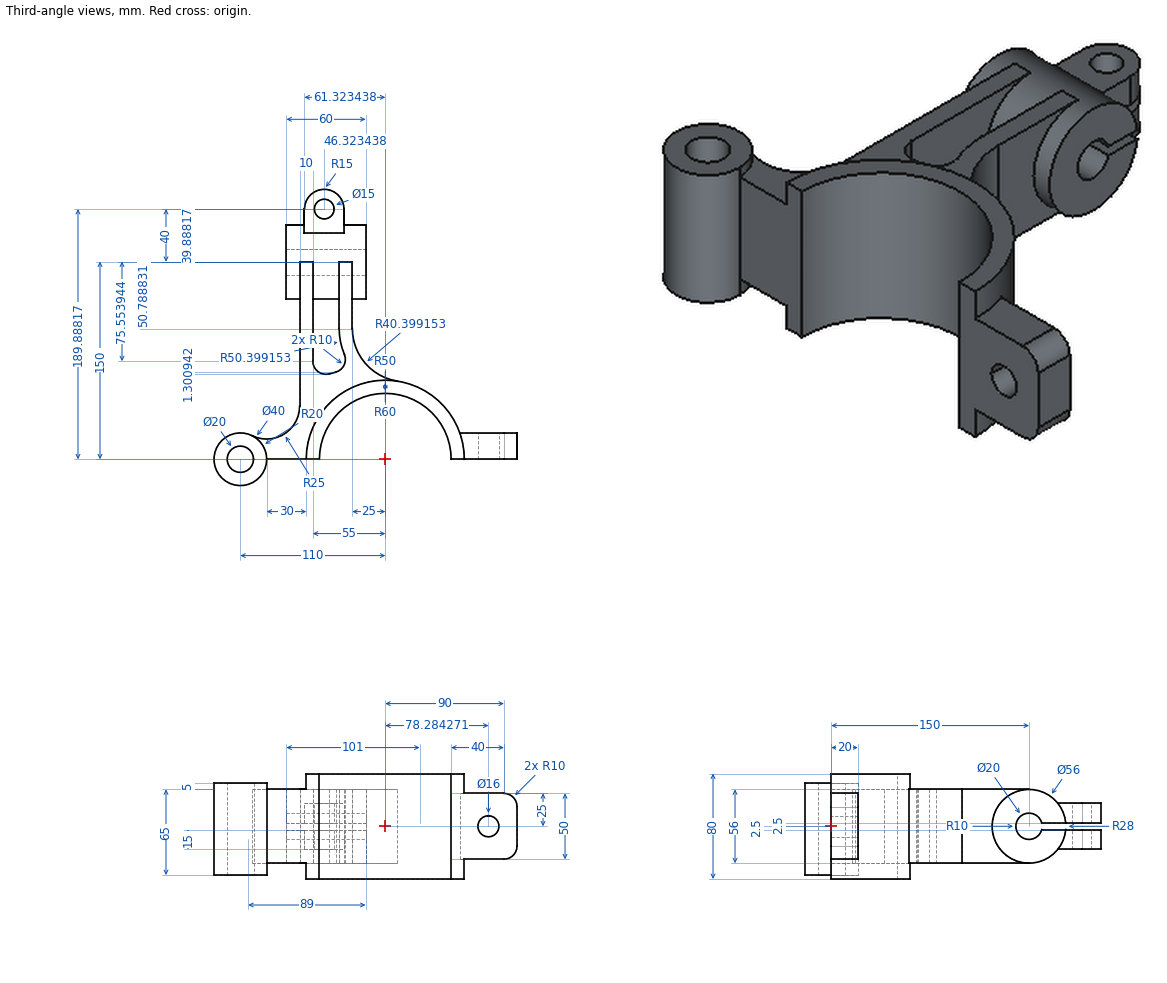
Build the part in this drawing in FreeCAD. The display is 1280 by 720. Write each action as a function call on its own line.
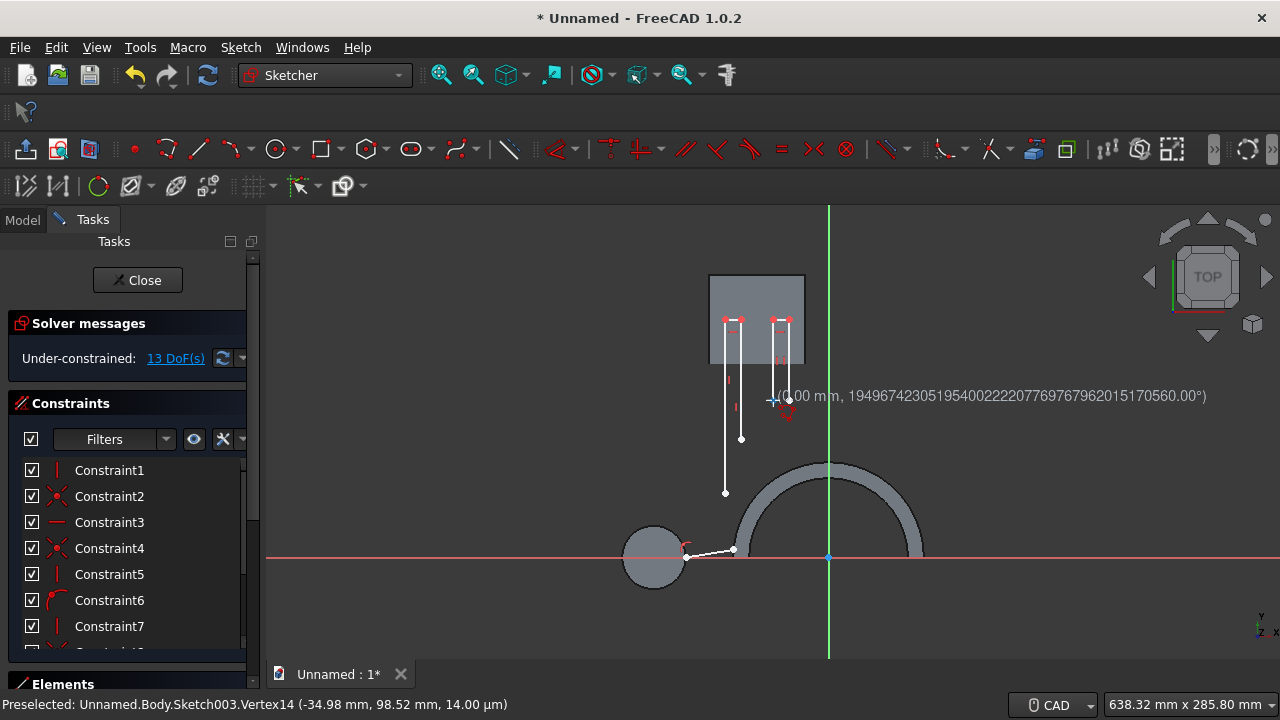
click(200, 150)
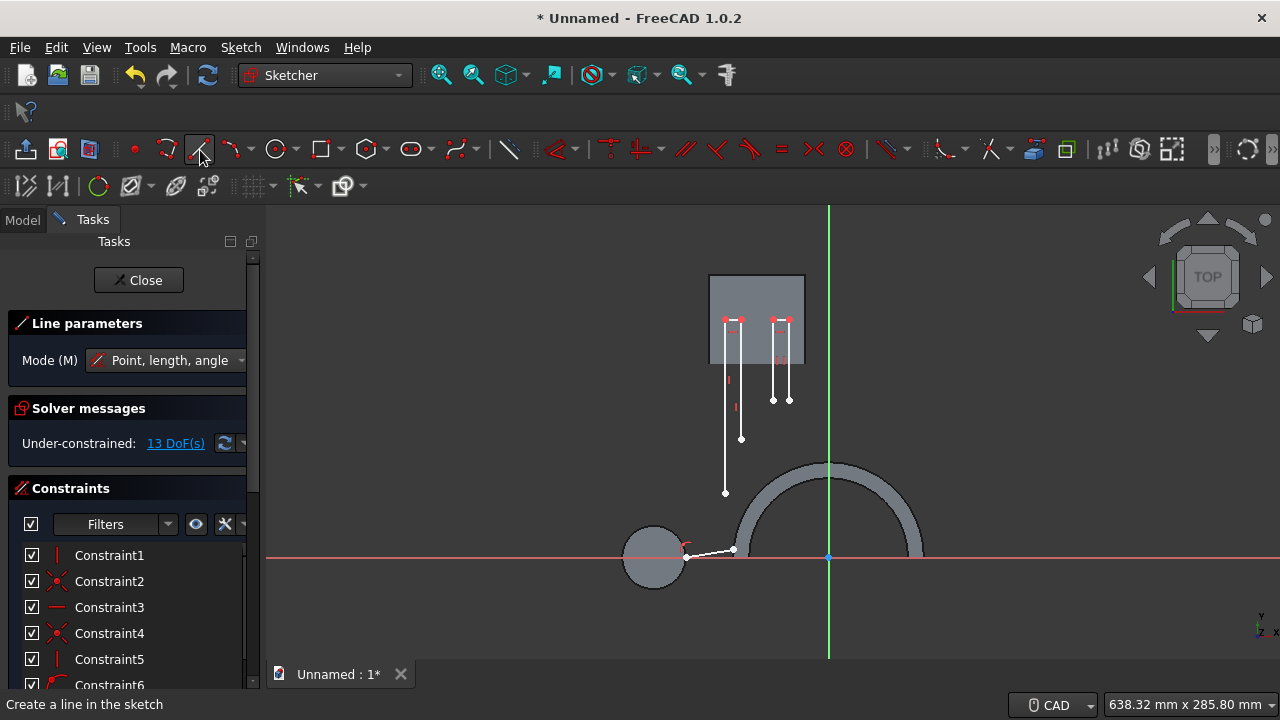
click(769, 452)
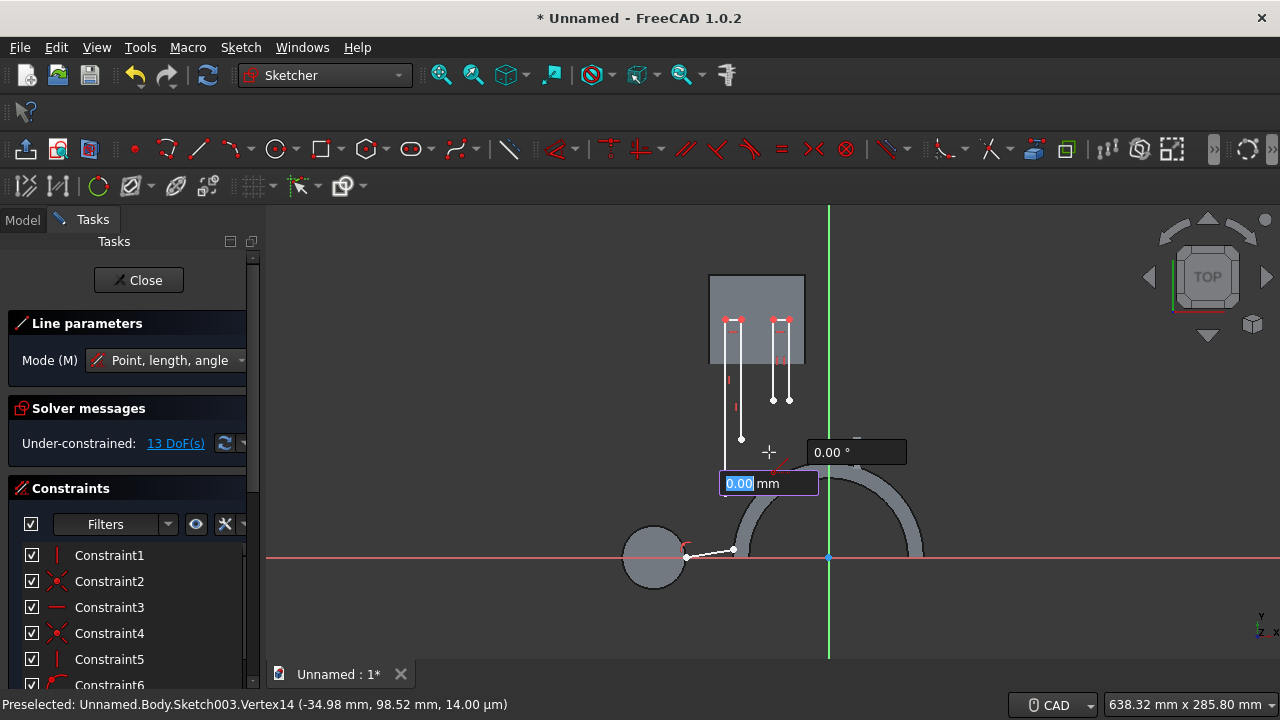
scroll(761, 455, up, 4)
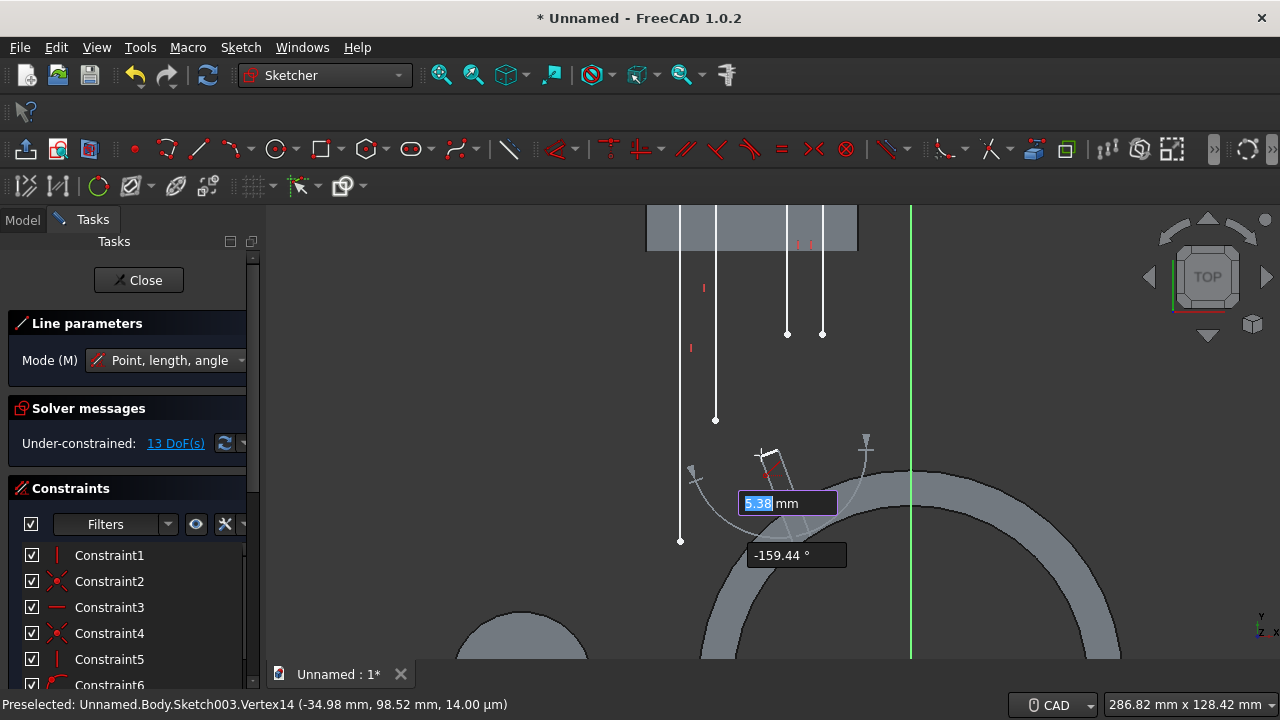
click(761, 453)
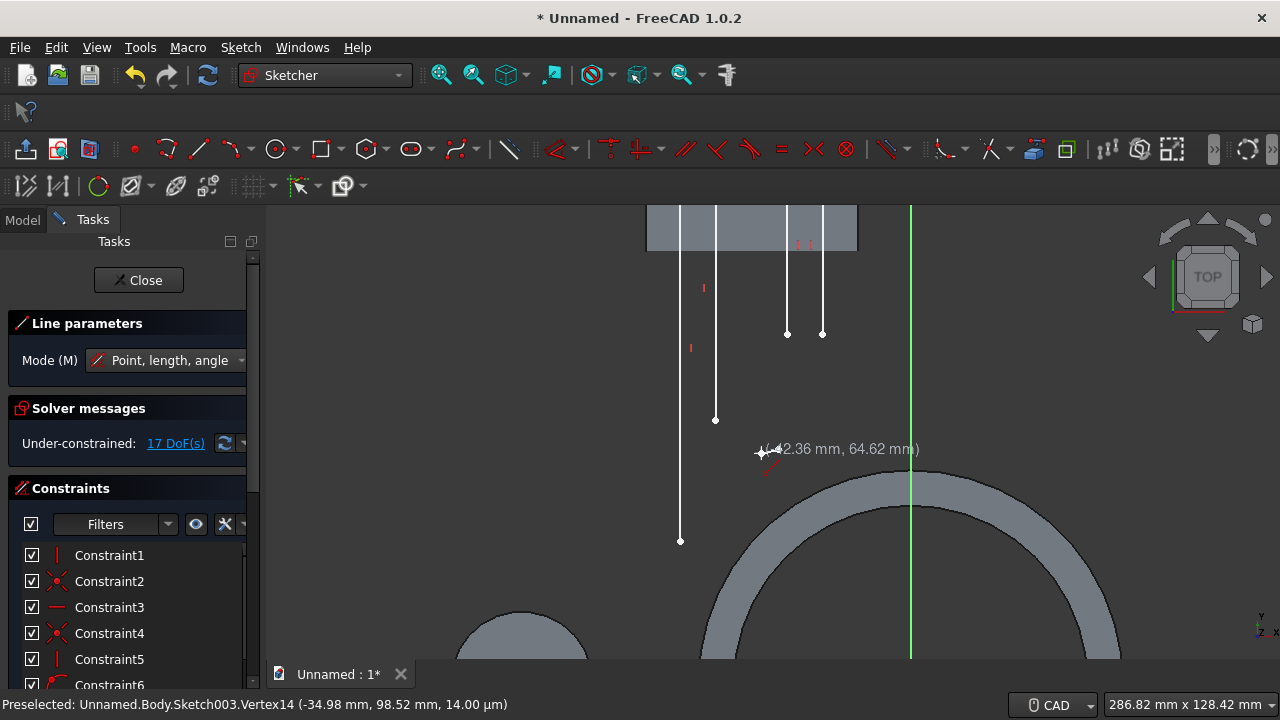
key(g)
key(3)
key(a)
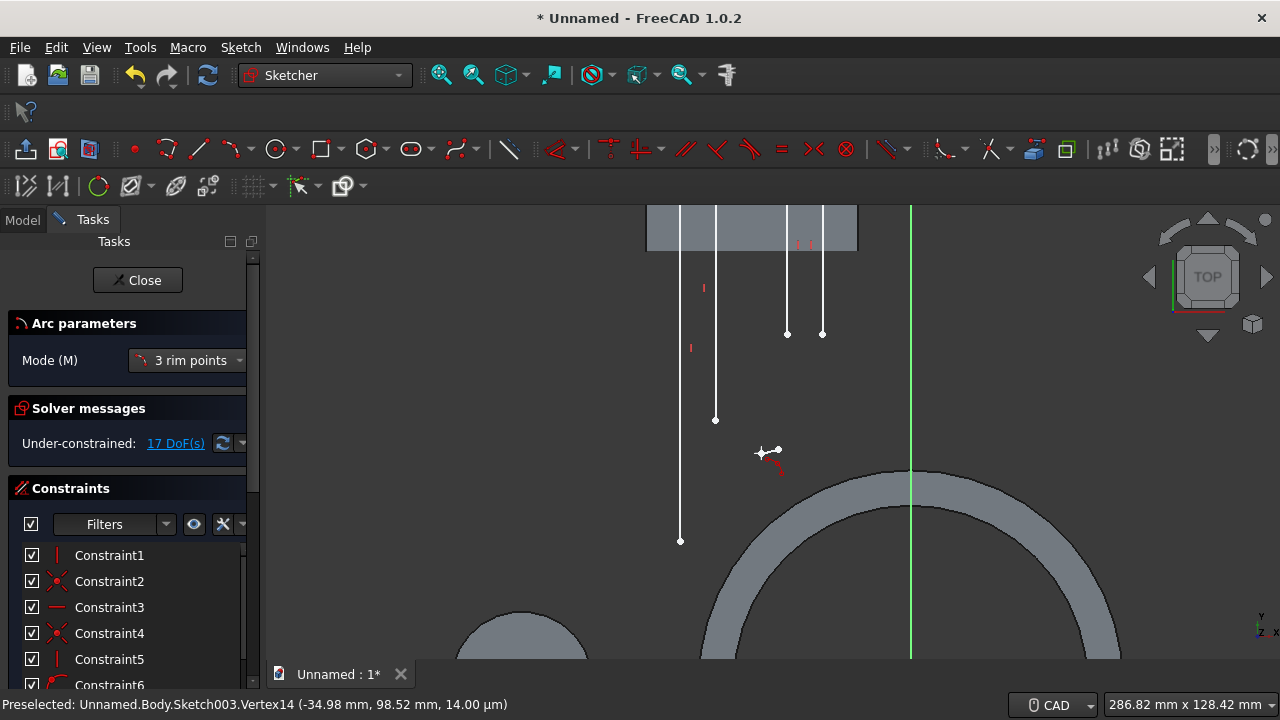
click(680, 541)
click(553, 619)
click(639, 615)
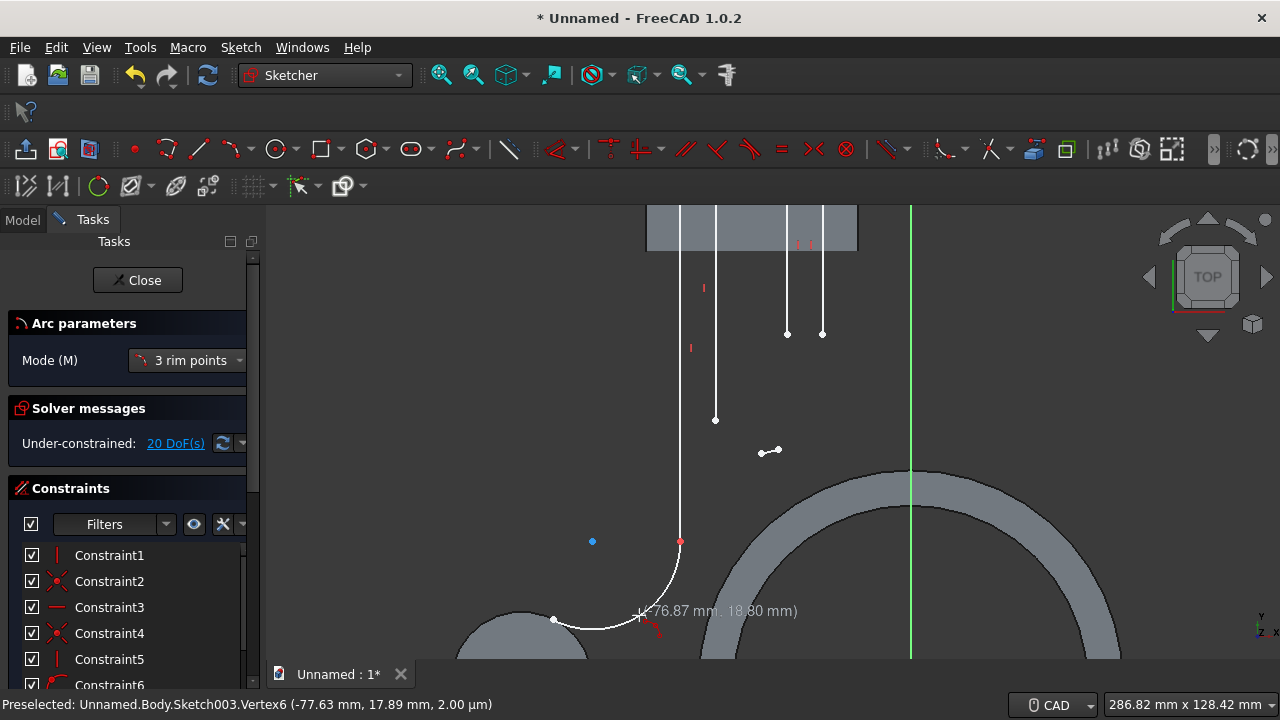
click(553, 620)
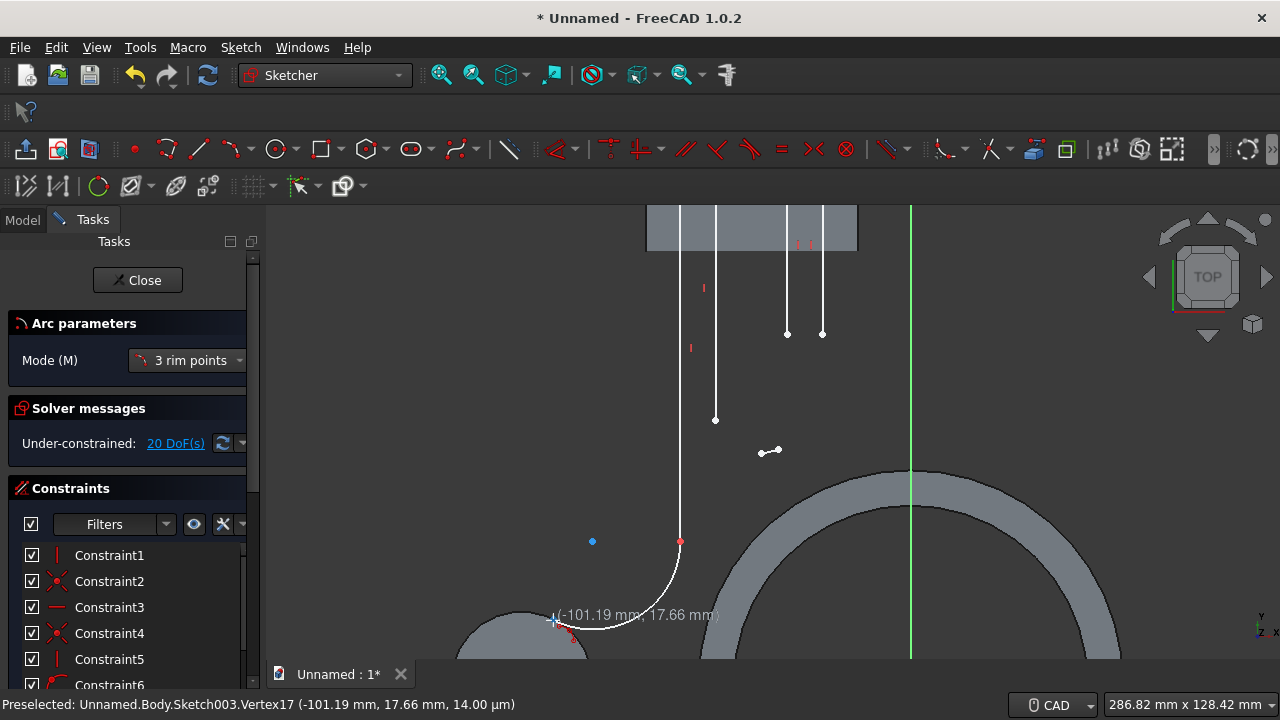
scroll(651, 450, down, 3)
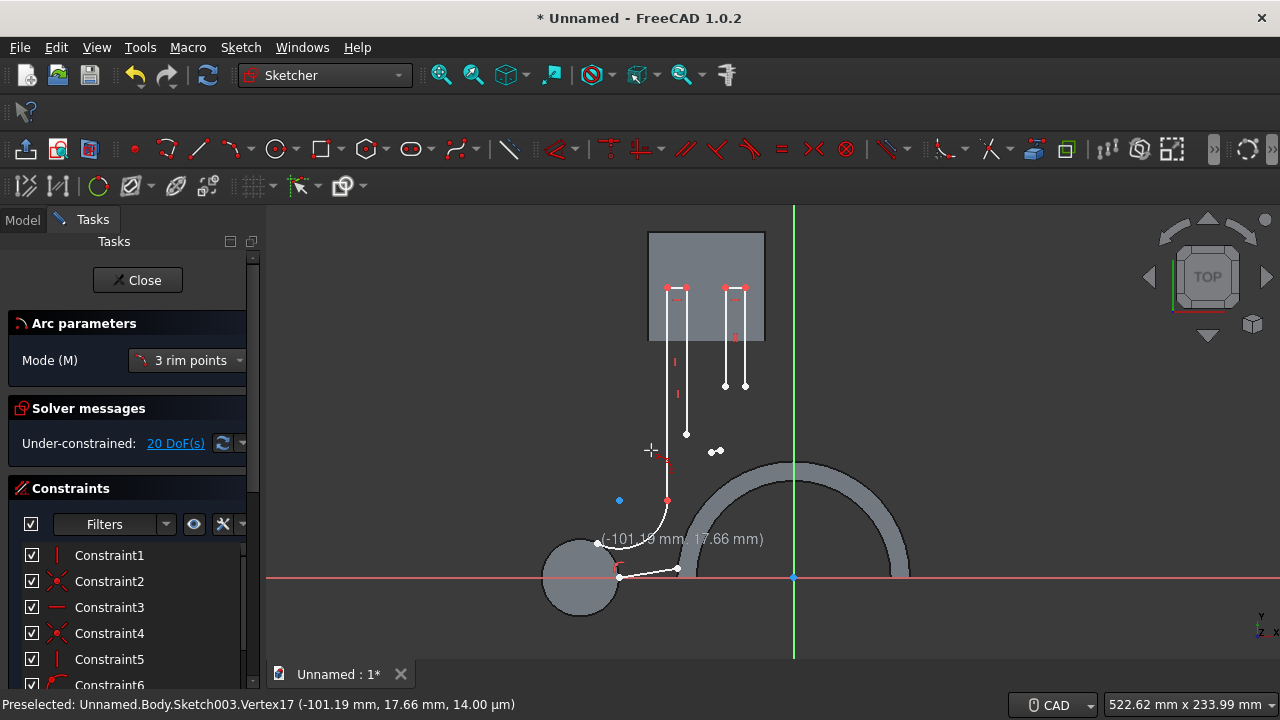
click(620, 578)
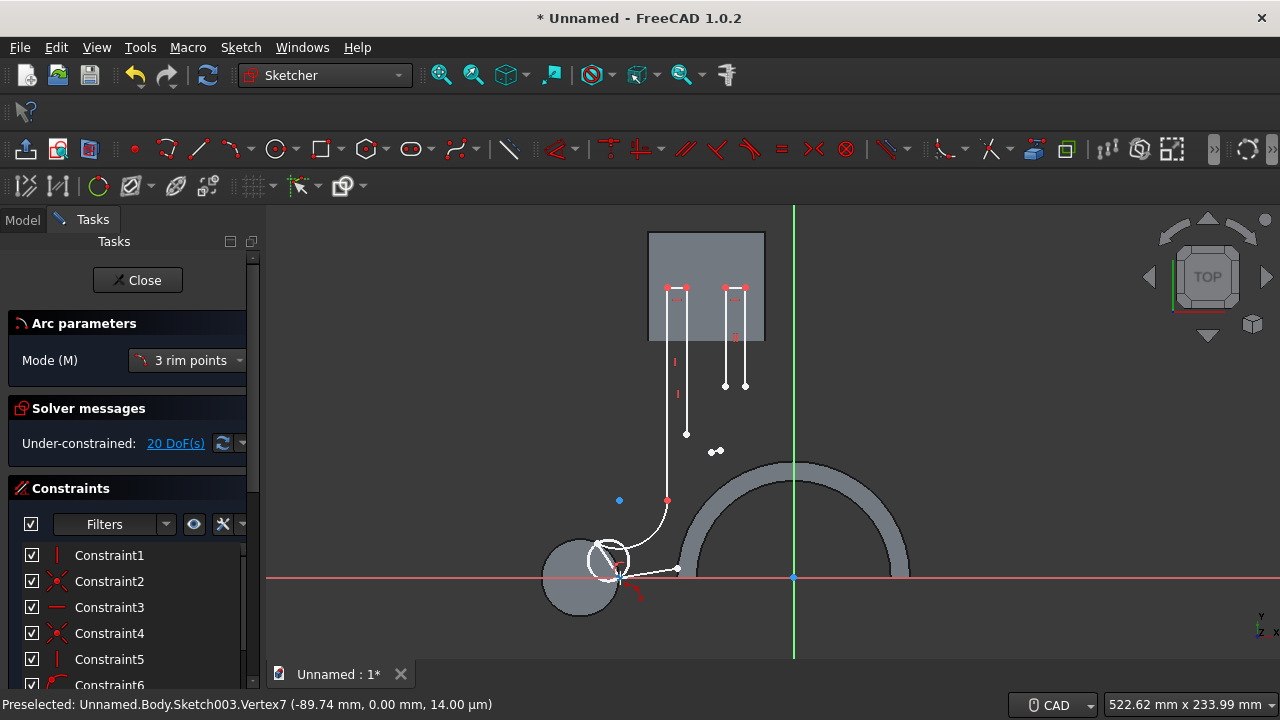
scroll(613, 557, up, 6)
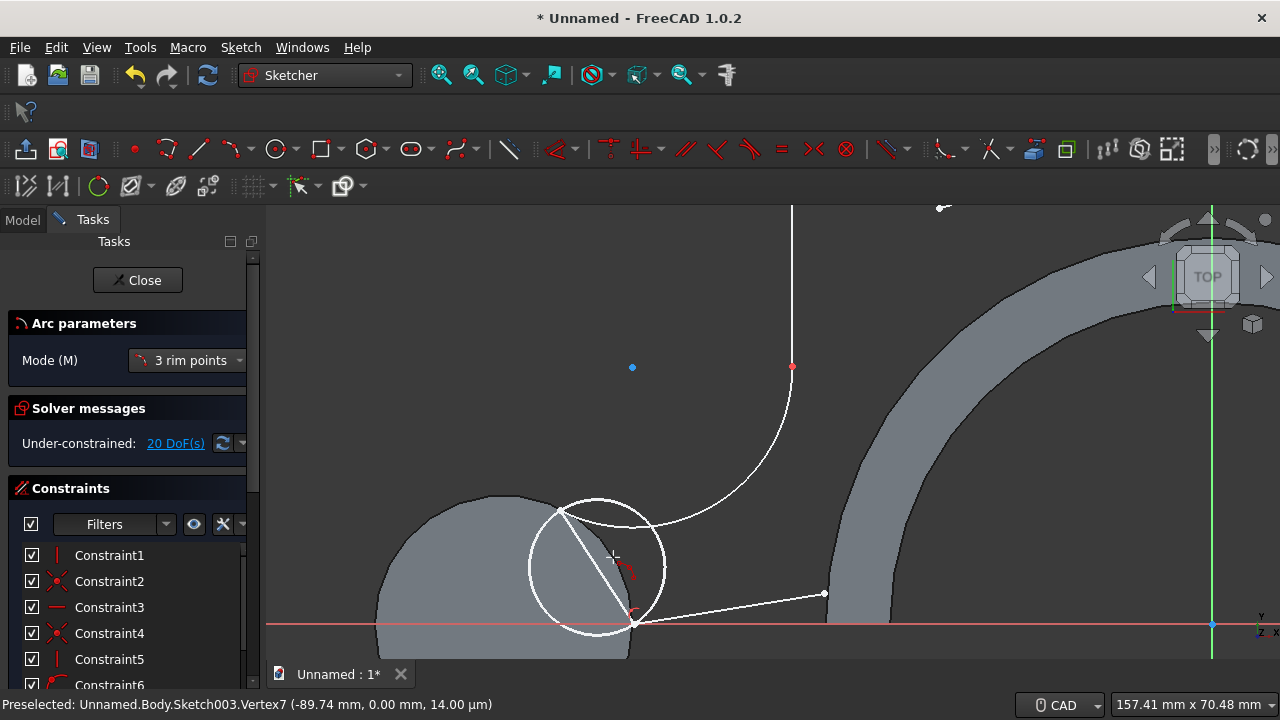
click(613, 556)